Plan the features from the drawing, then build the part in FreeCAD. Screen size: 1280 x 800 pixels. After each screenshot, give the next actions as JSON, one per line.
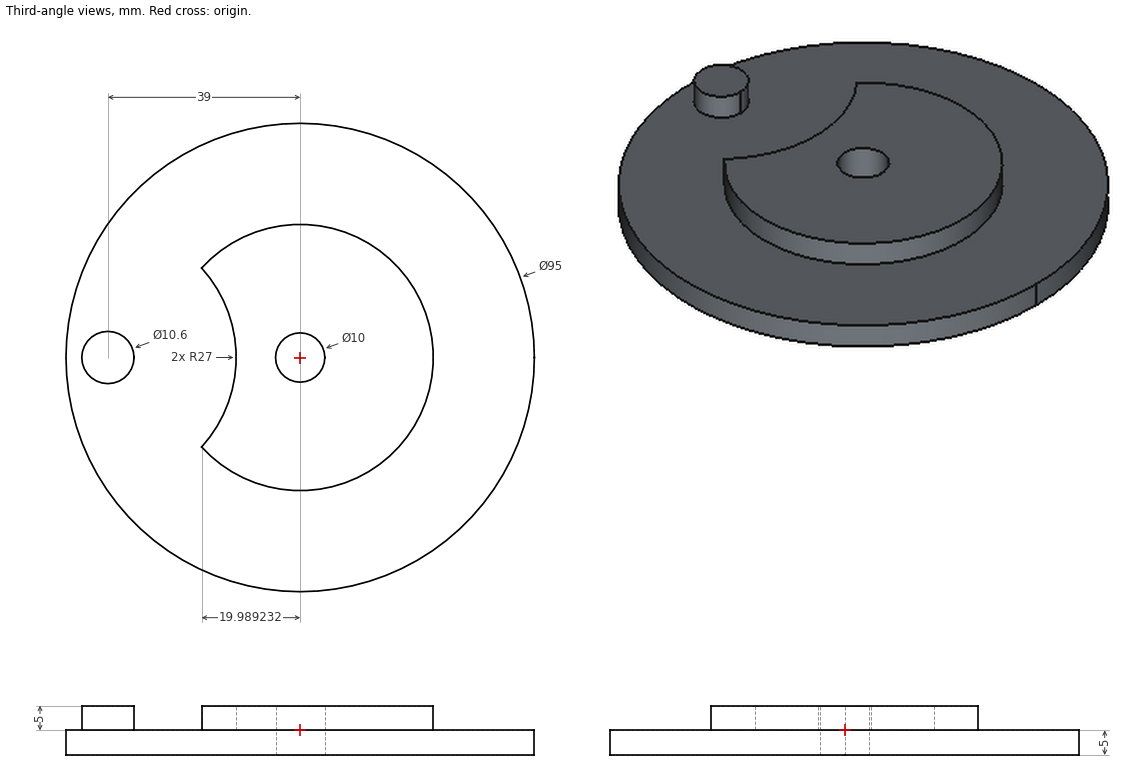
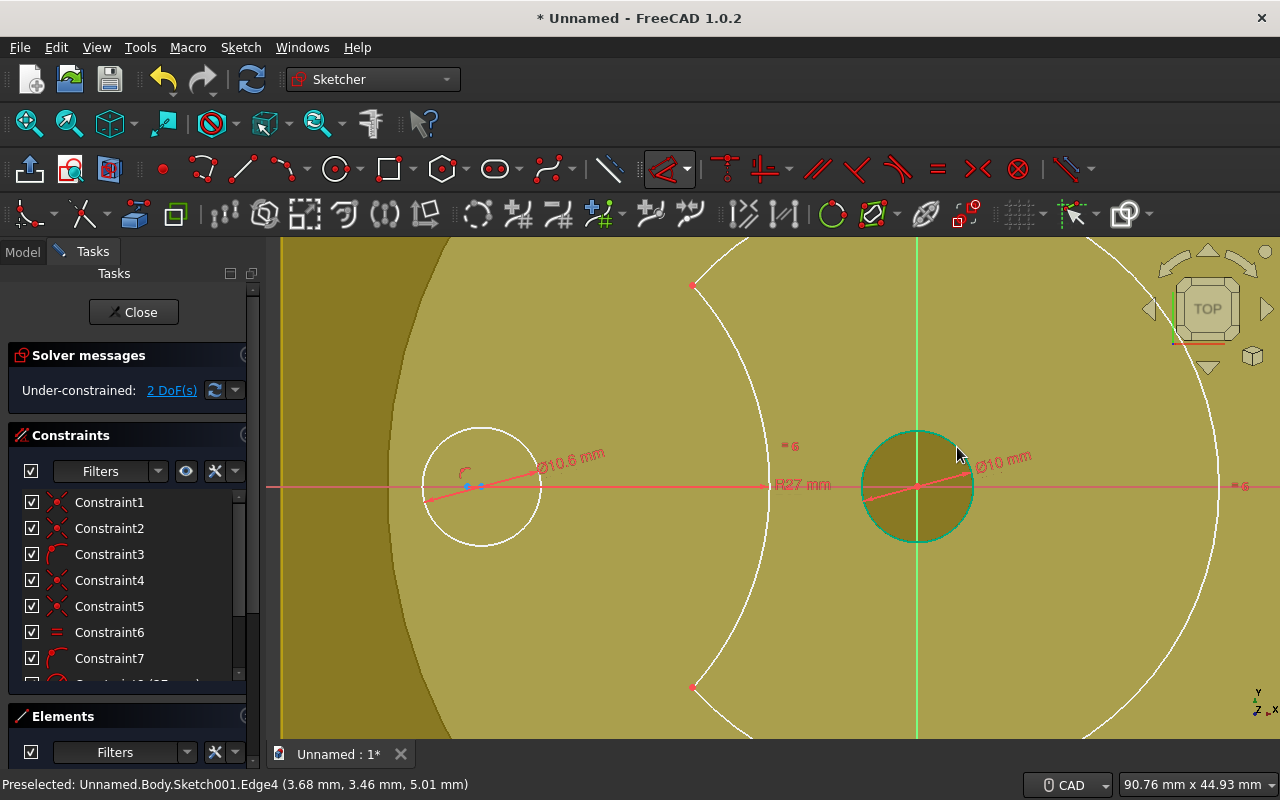
{"action": "left_click", "coordinate": [482, 487]}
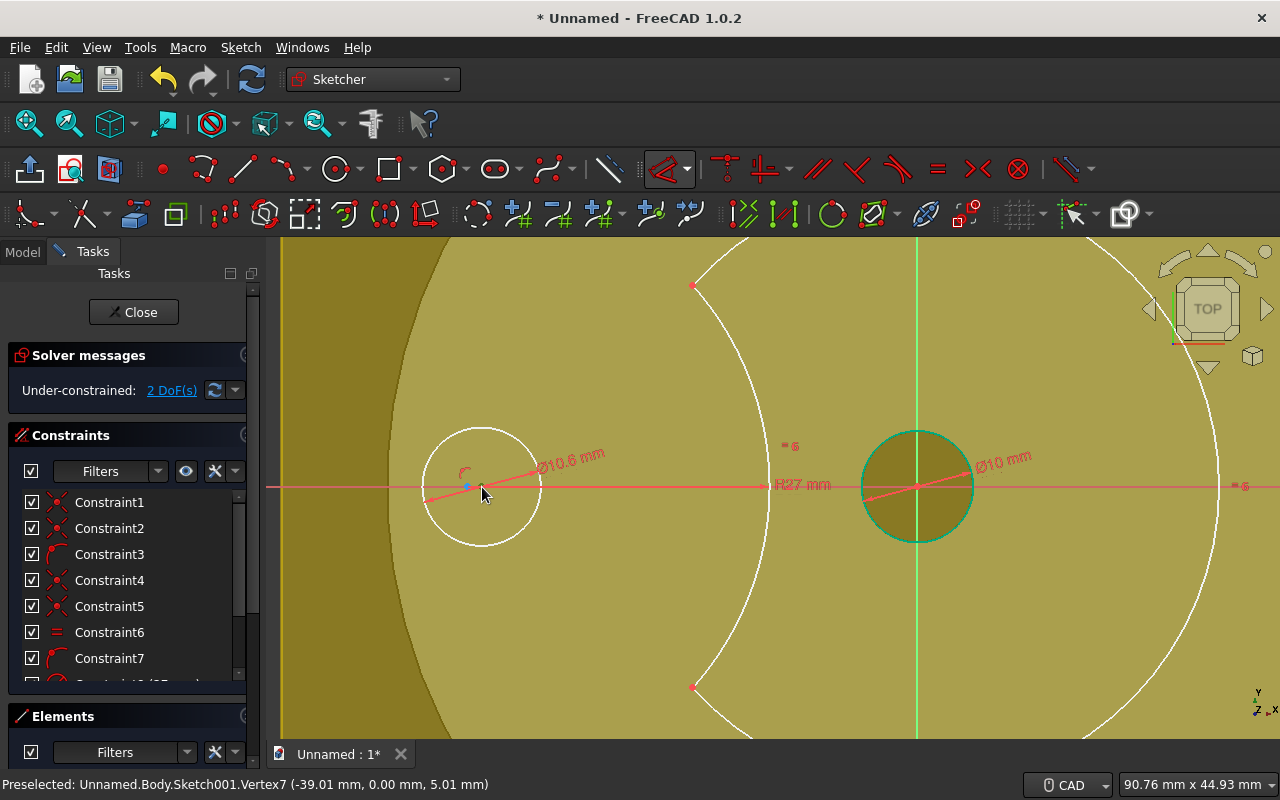
{"action": "left_click", "coordinate": [690, 170]}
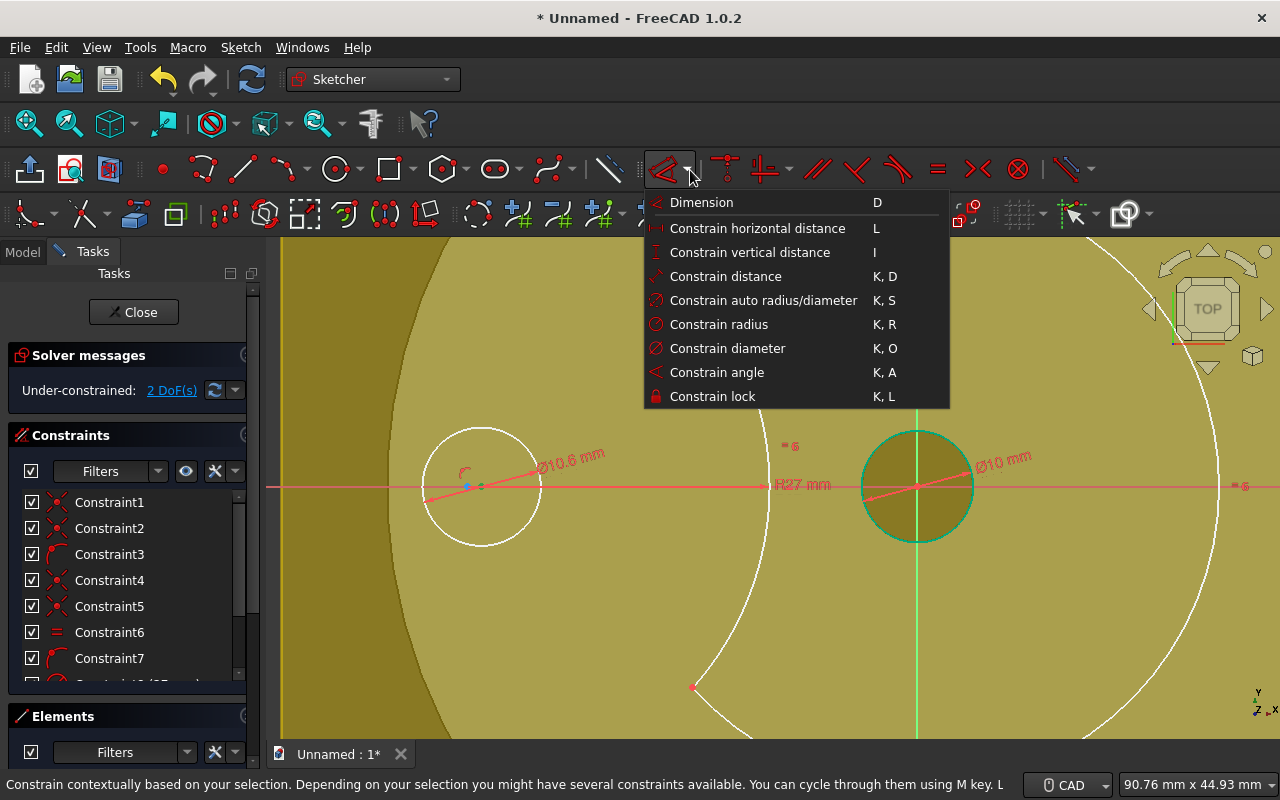
{"action": "left_click", "coordinate": [797, 228]}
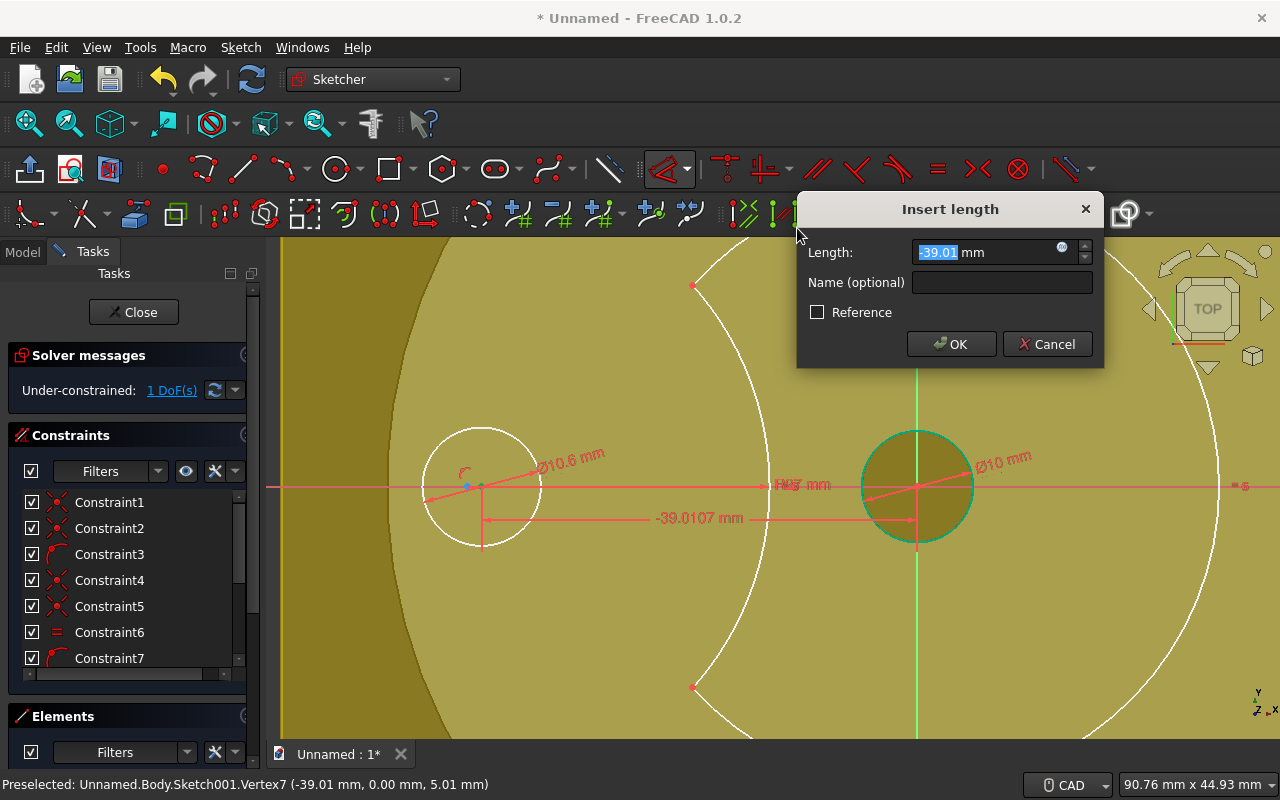
{"action": "type", "text": "-39"}
{"action": "key", "text": "Return"}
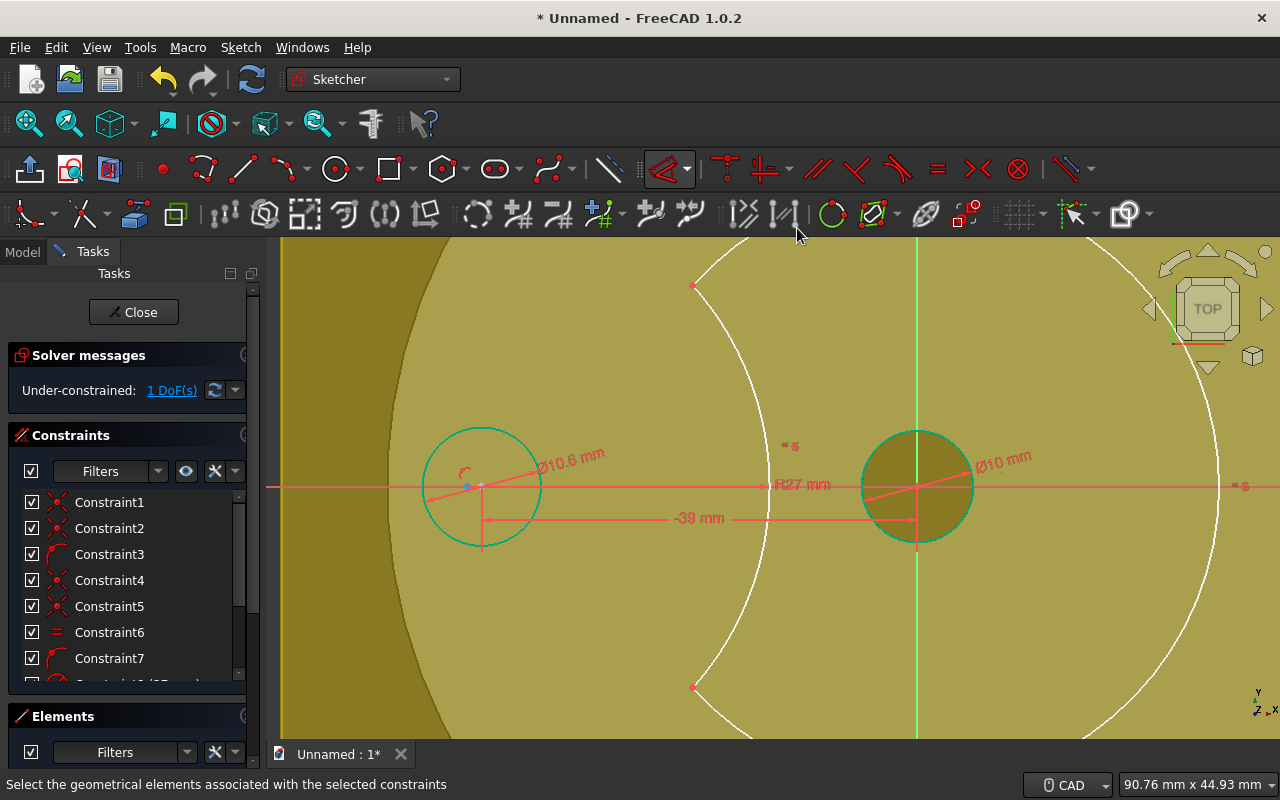
{"action": "left_click", "coordinate": [693, 688]}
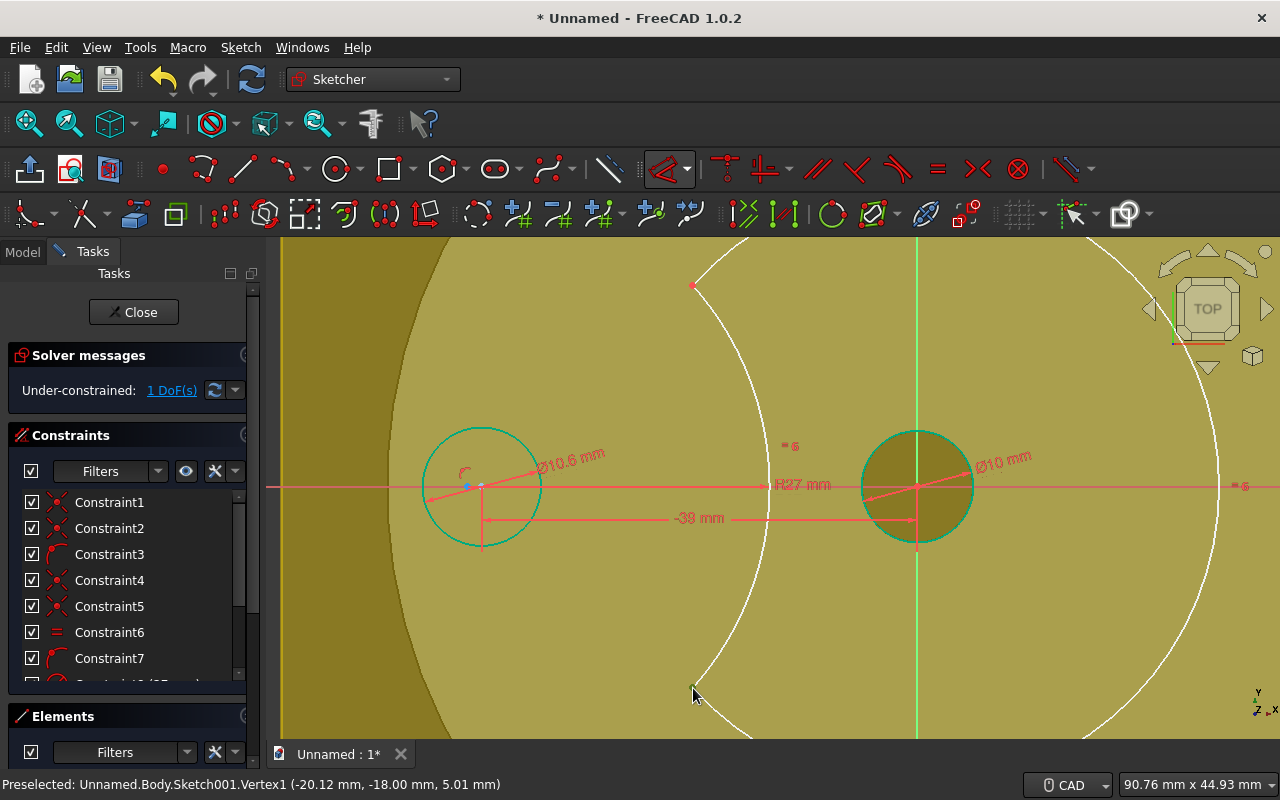
{"action": "key", "text": "l"}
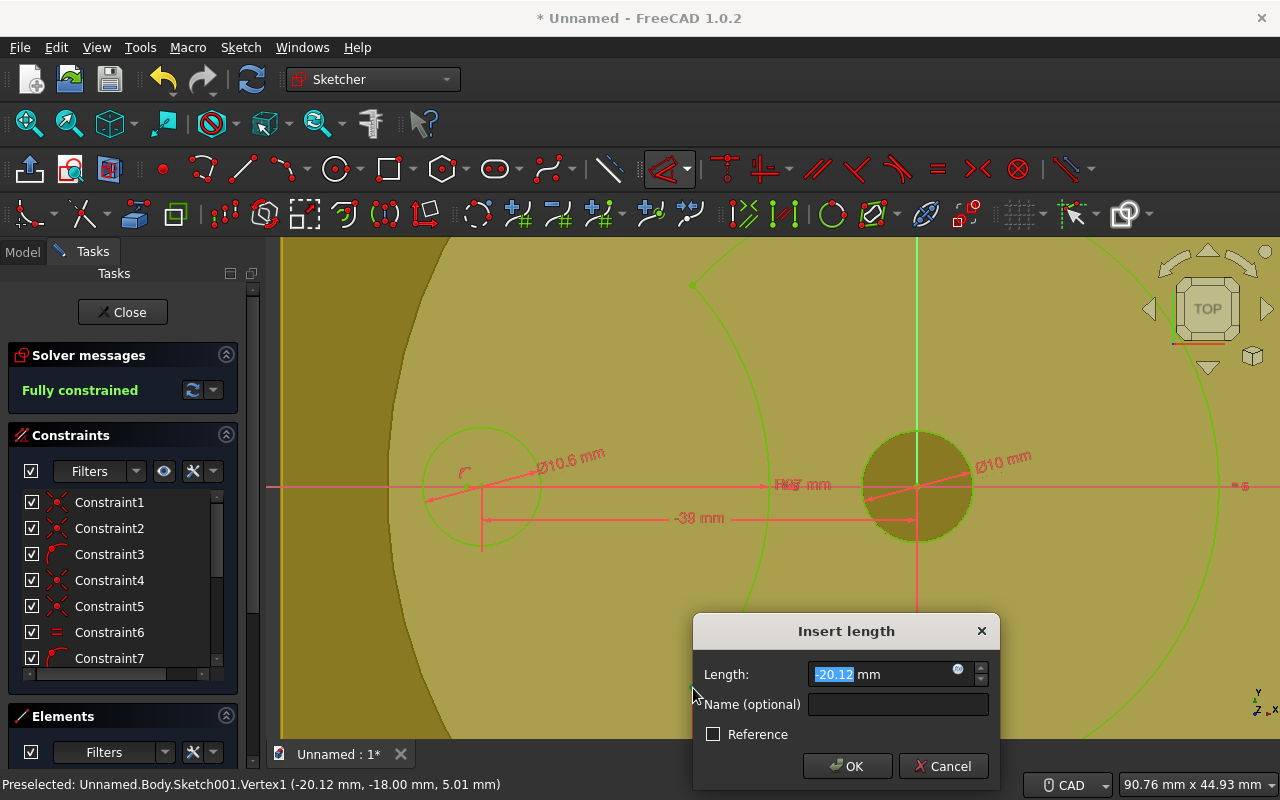
{"action": "type", "text": "-19.989232"}
{"action": "key", "text": "Return"}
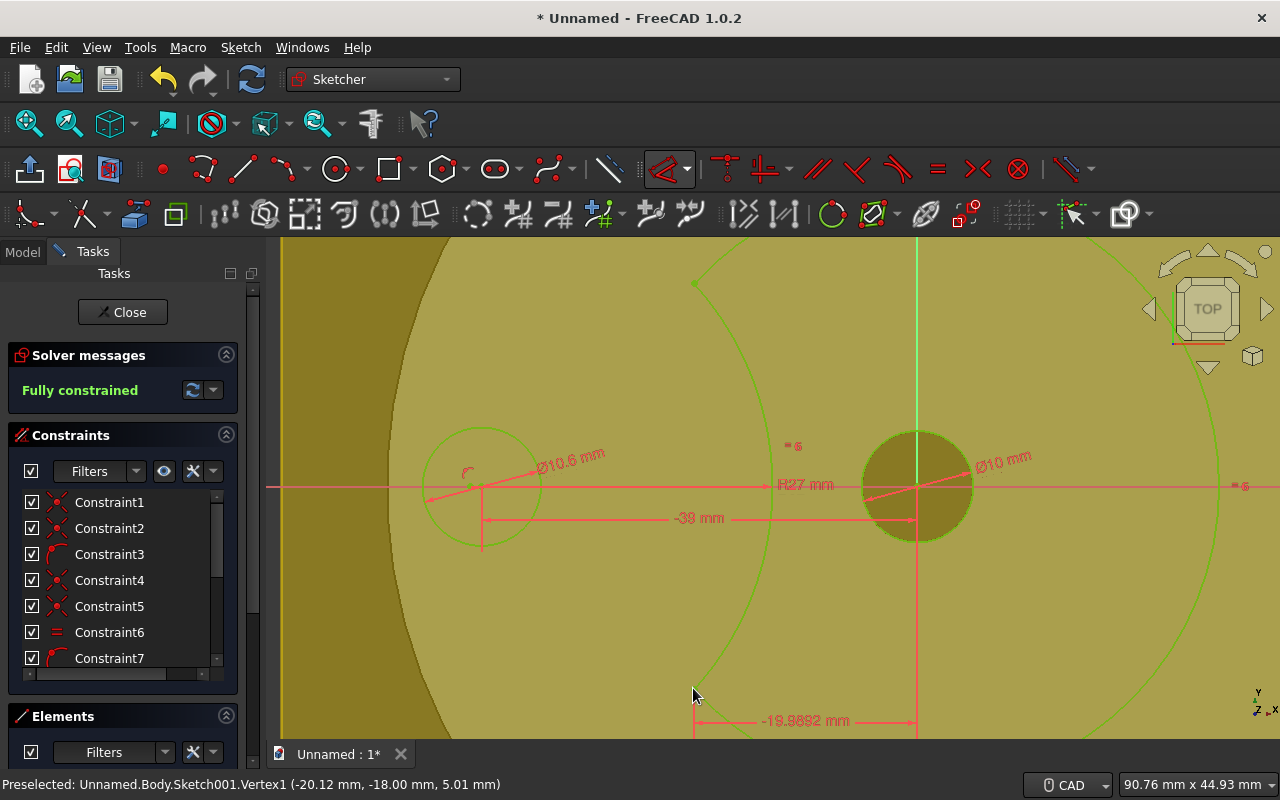
{"action": "left_click", "coordinate": [123, 312]}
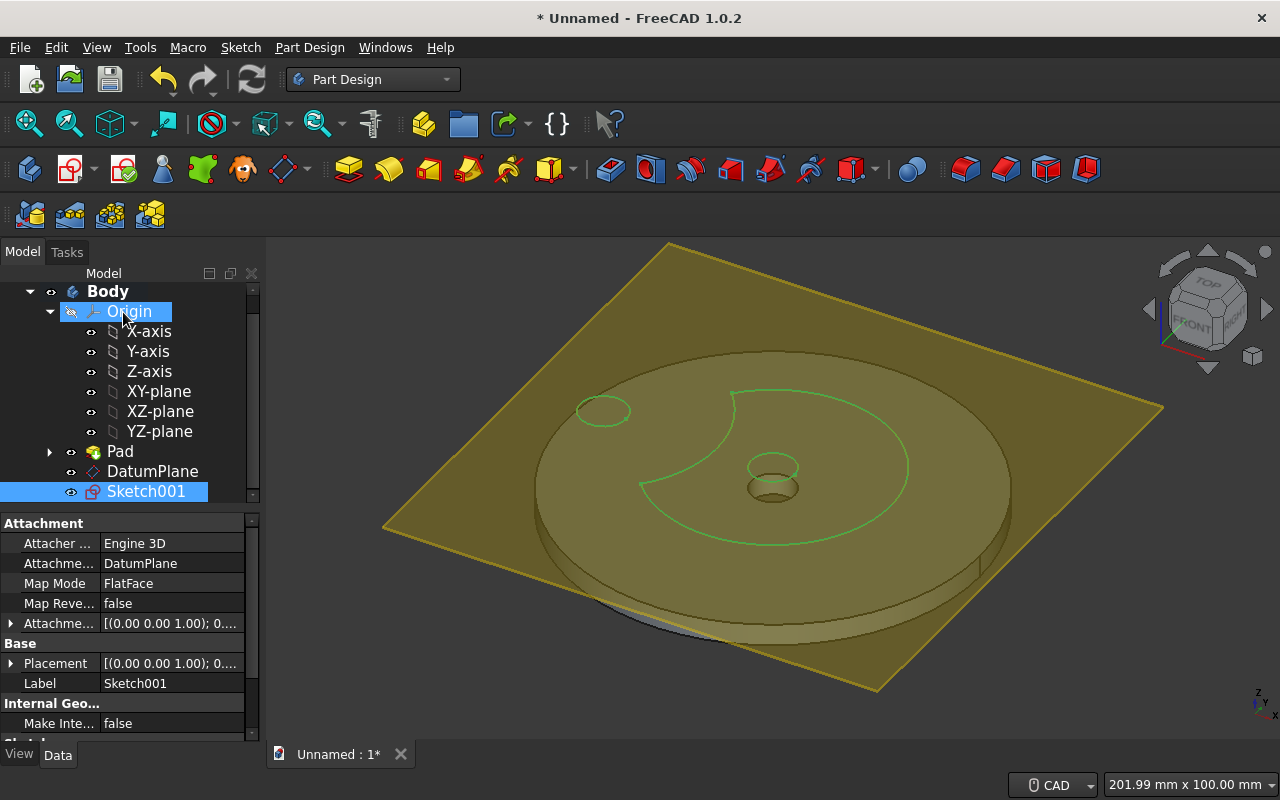
{"action": "left_click", "coordinate": [350, 170]}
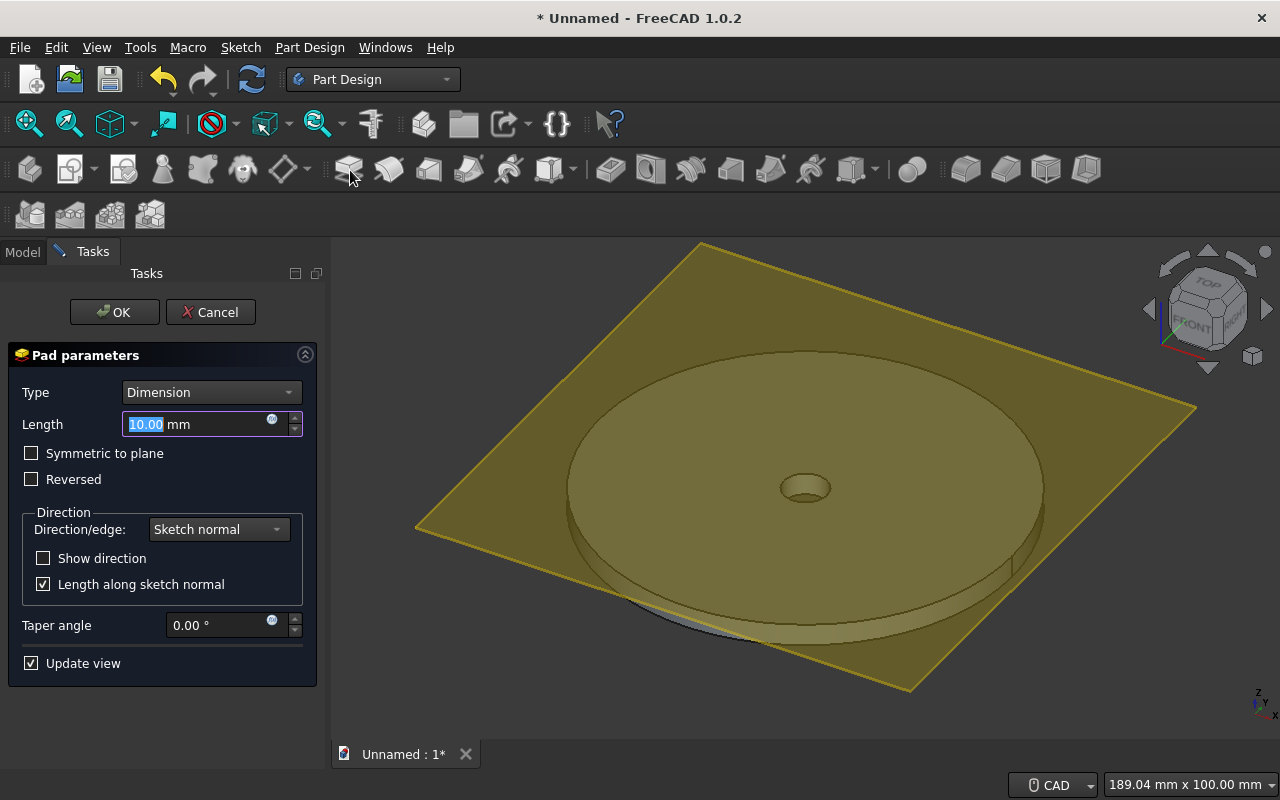
{"action": "type", "text": "5"}
{"action": "key", "text": "Tab"}